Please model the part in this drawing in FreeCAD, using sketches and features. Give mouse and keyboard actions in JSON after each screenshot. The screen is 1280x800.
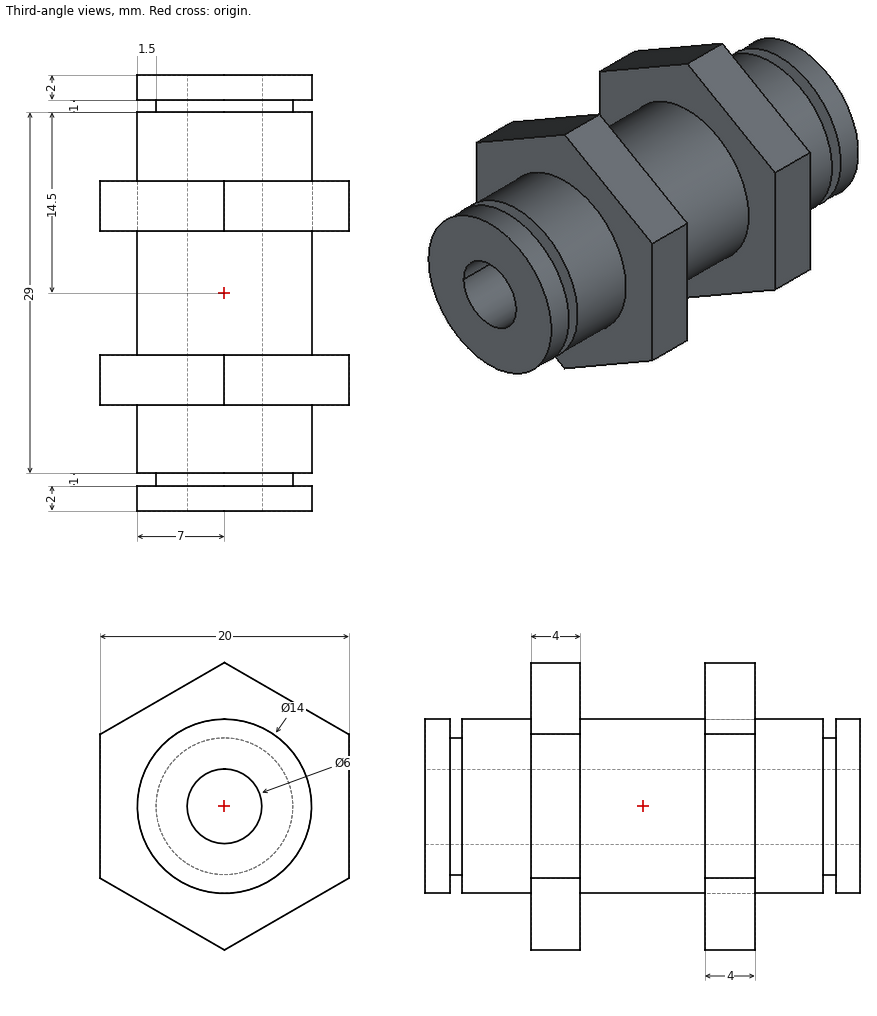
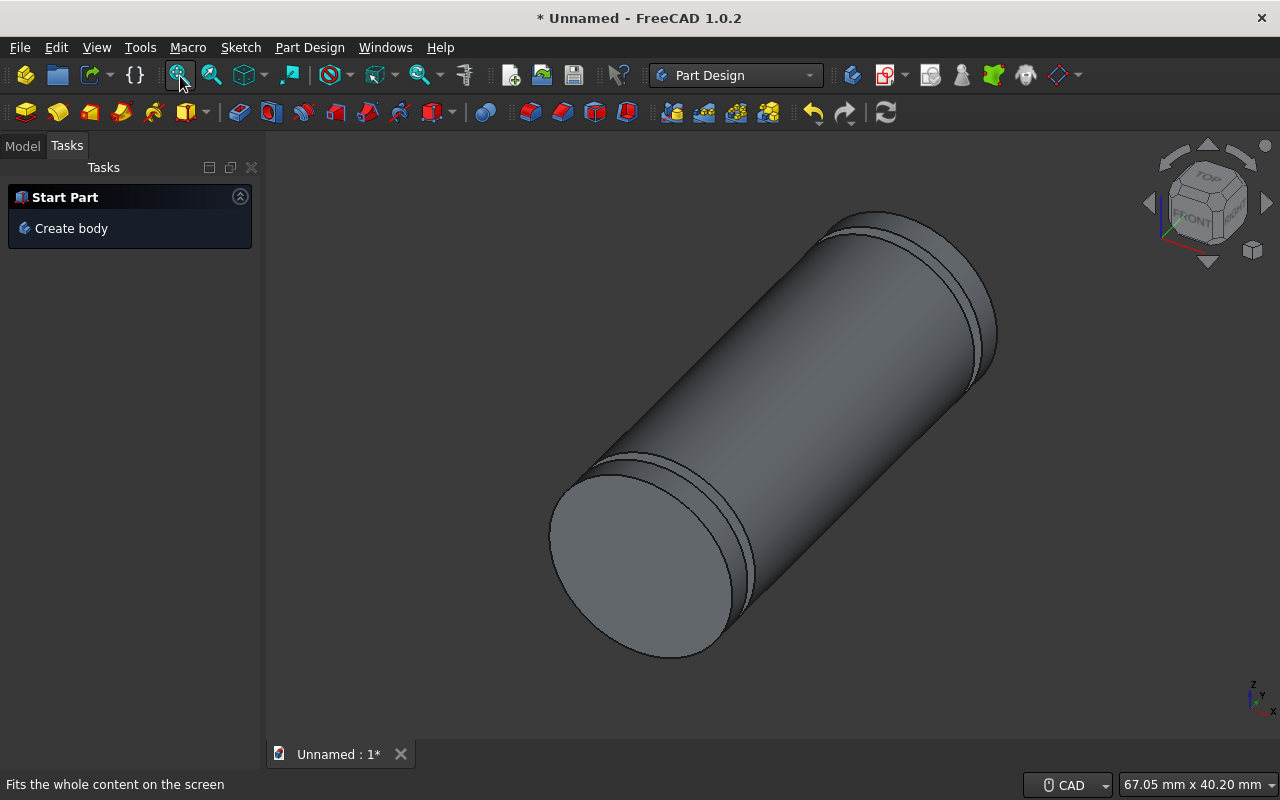
{"action": "key", "text": "4"}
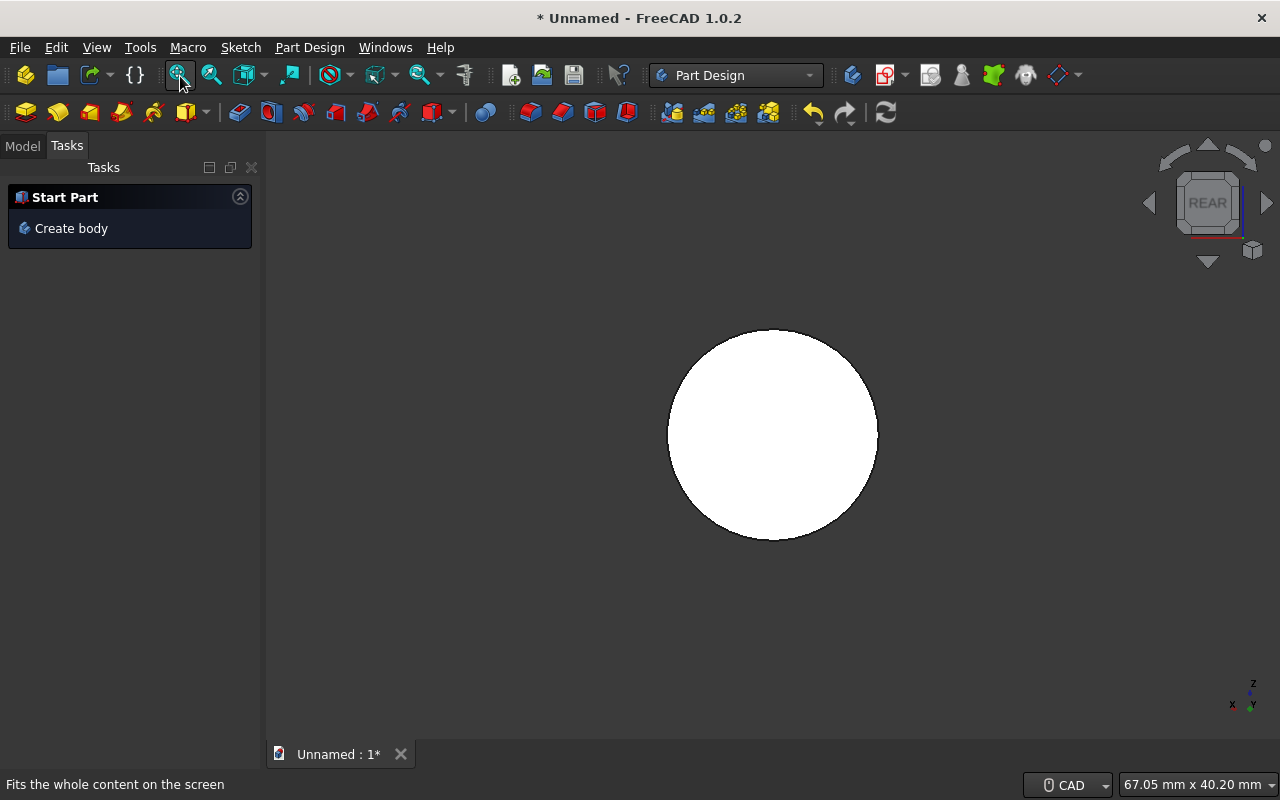
{"action": "left_click", "coordinate": [180, 76]}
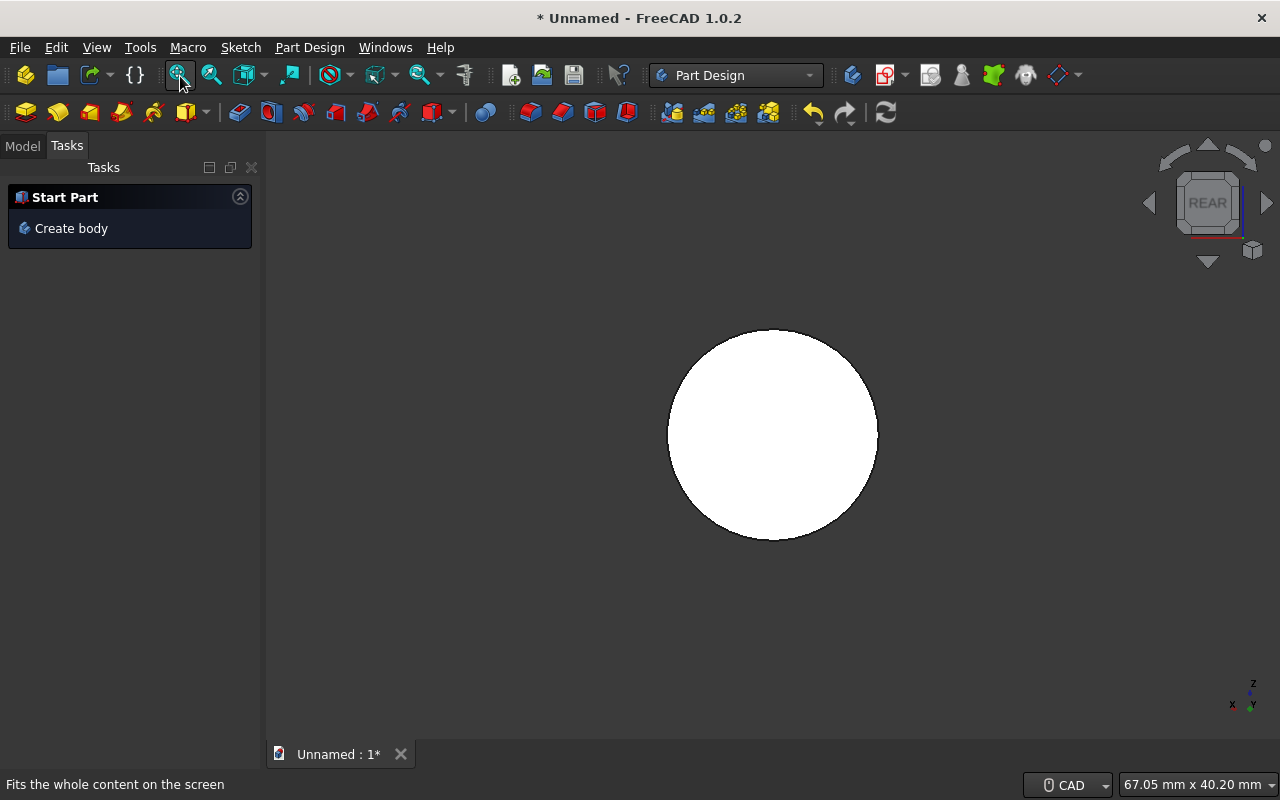
{"action": "left_click", "coordinate": [773, 434]}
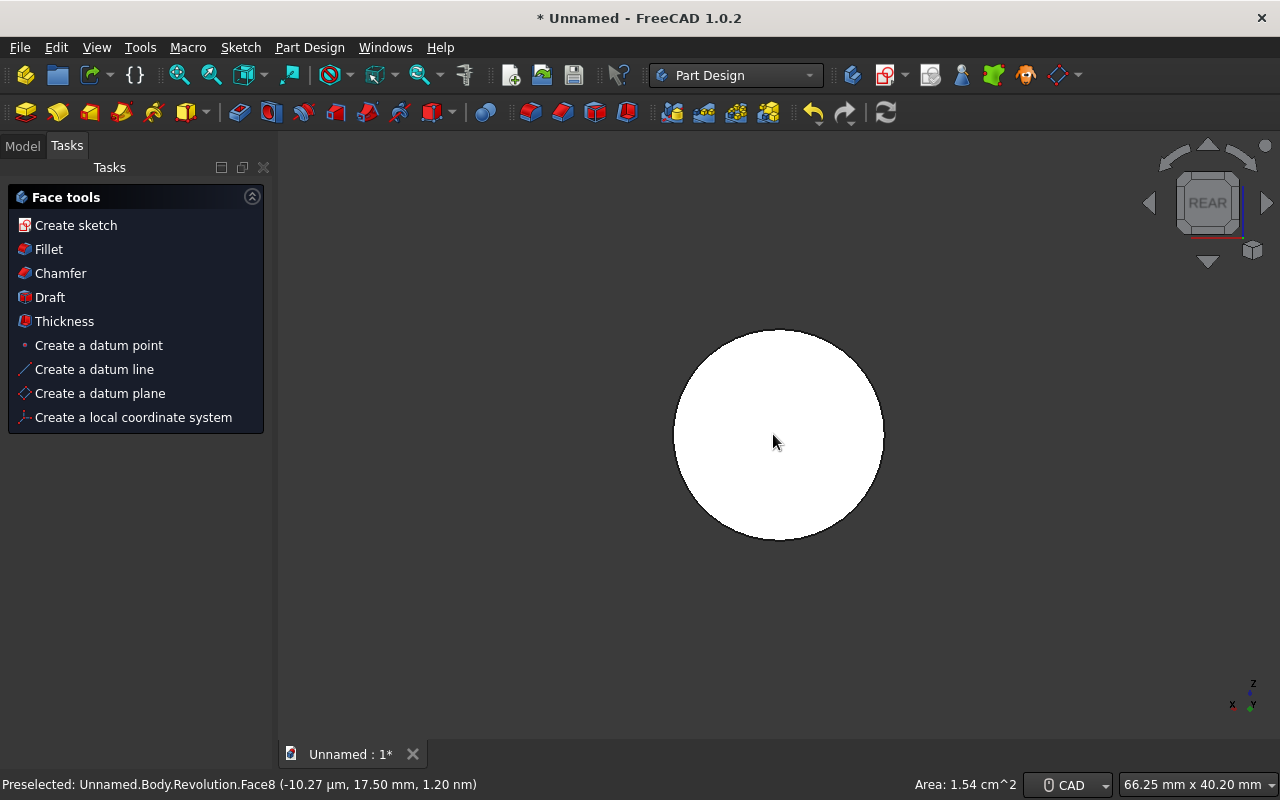
{"action": "left_click", "coordinate": [886, 76]}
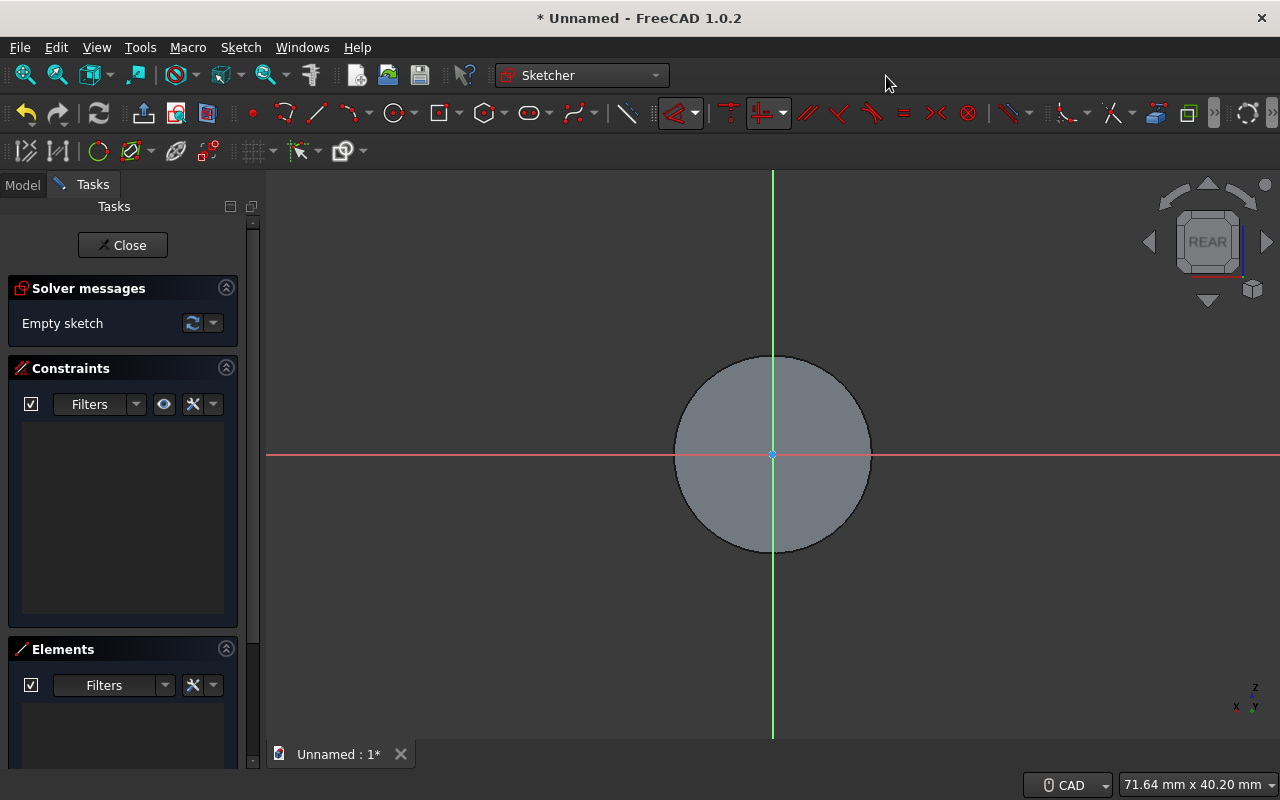
{"action": "scroll", "coordinate": [795, 455], "scroll_direction": "up", "scroll_amount": 7}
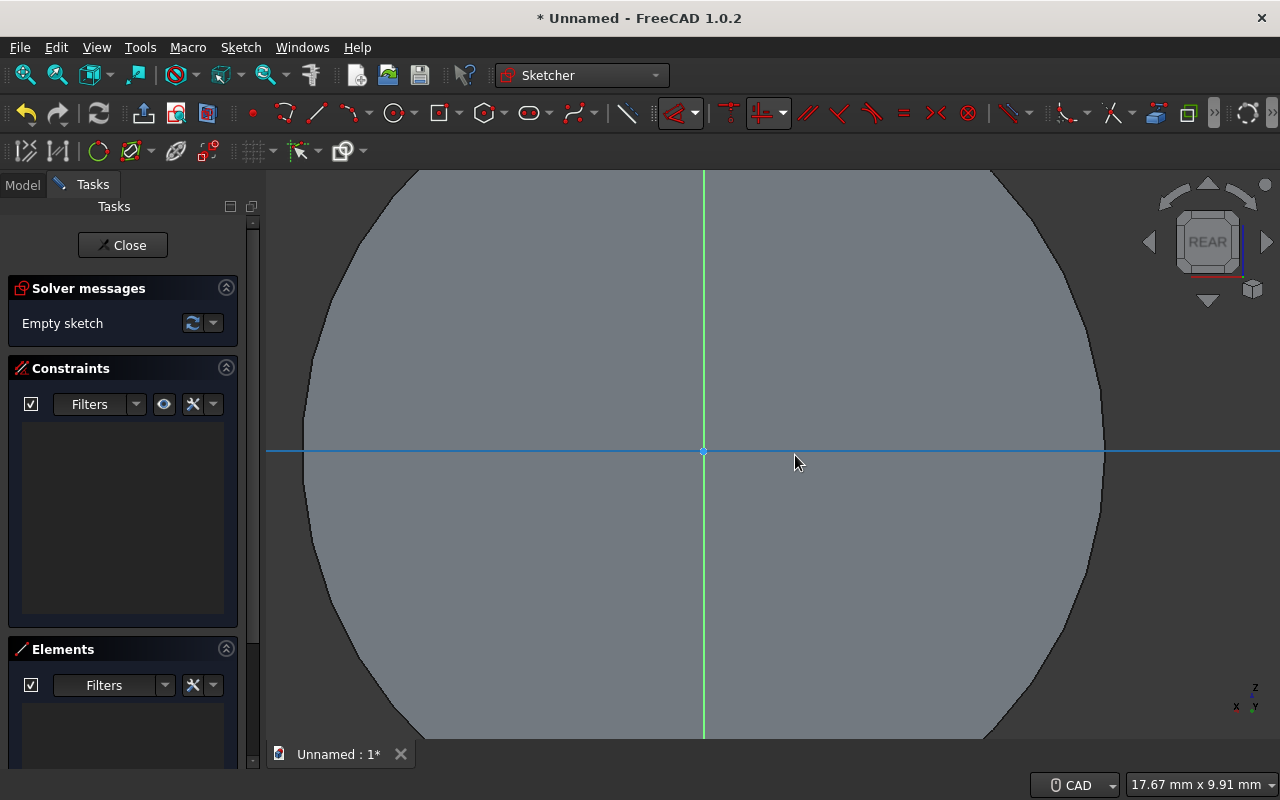
{"action": "left_click", "coordinate": [394, 114]}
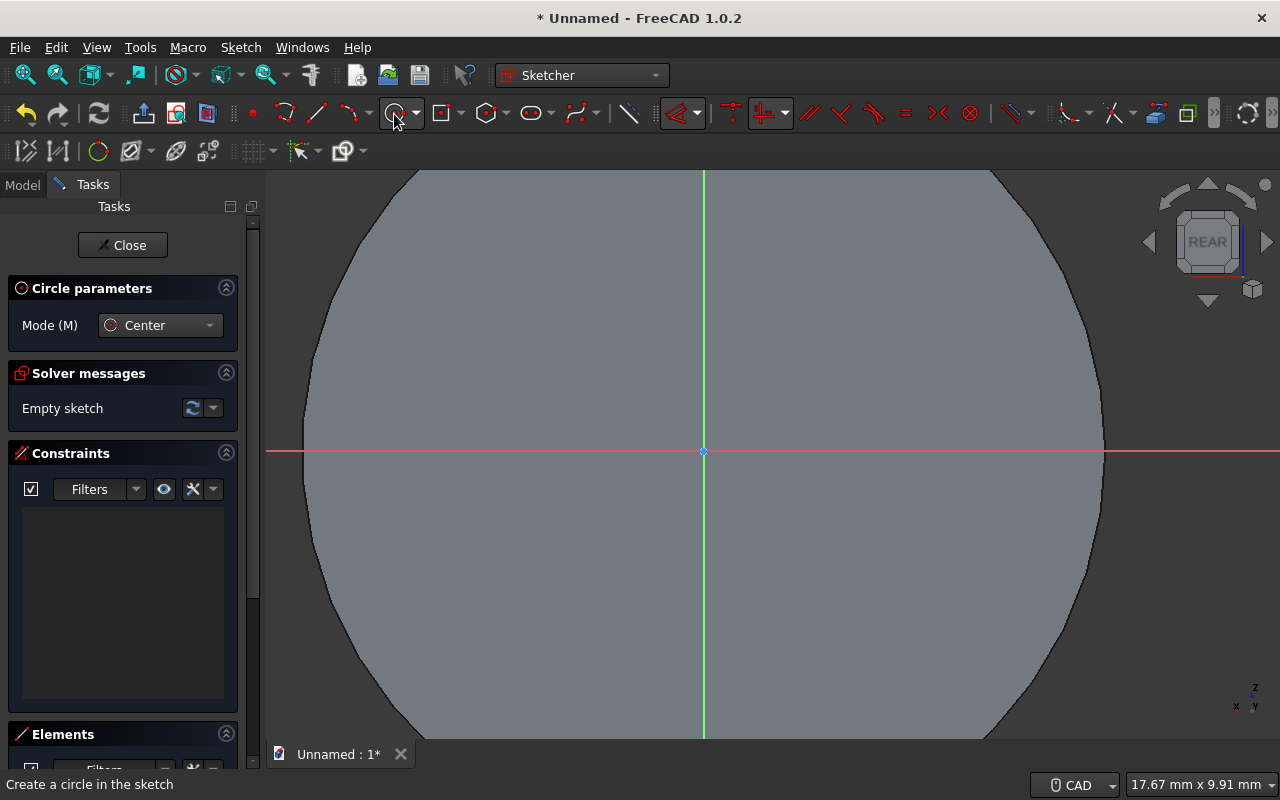
{"action": "left_click", "coordinate": [704, 451]}
{"action": "left_click", "coordinate": [825, 330]}
{"action": "key", "text": "Escape"}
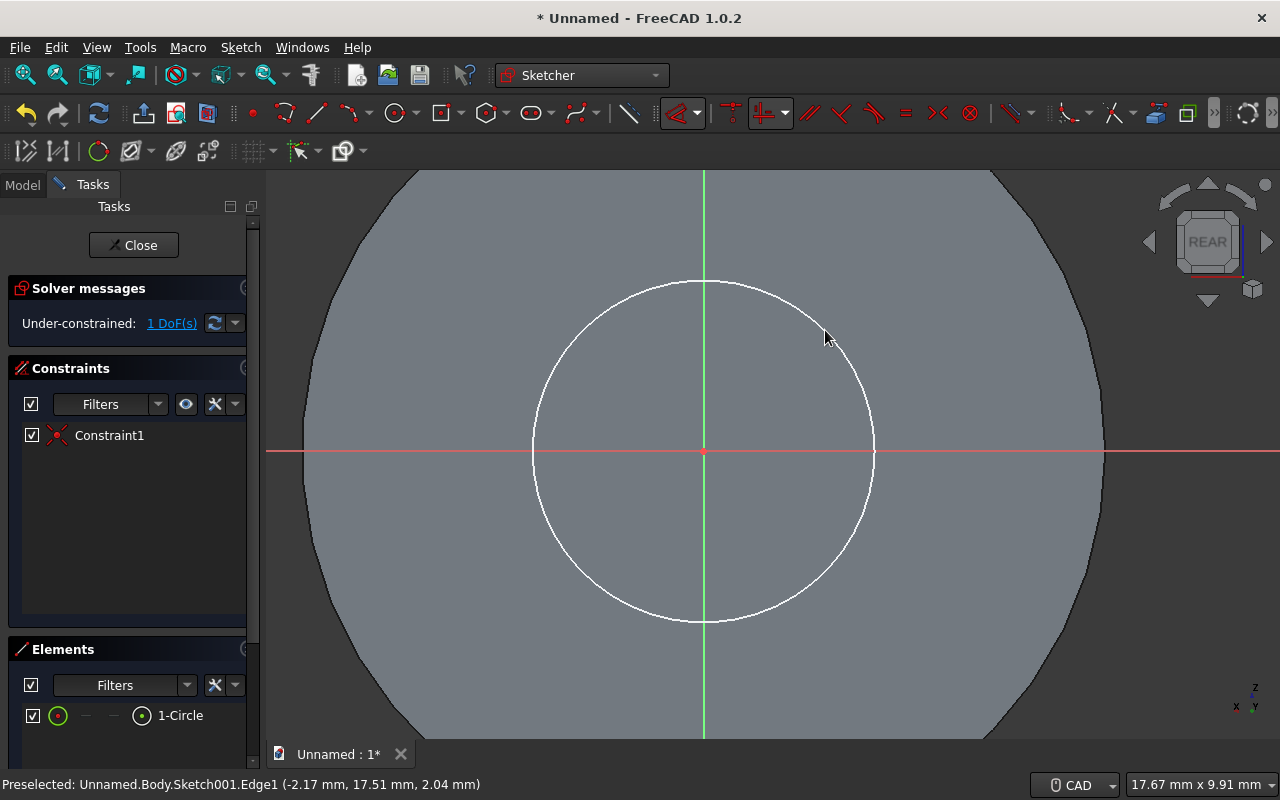
{"action": "left_click", "coordinate": [824, 330]}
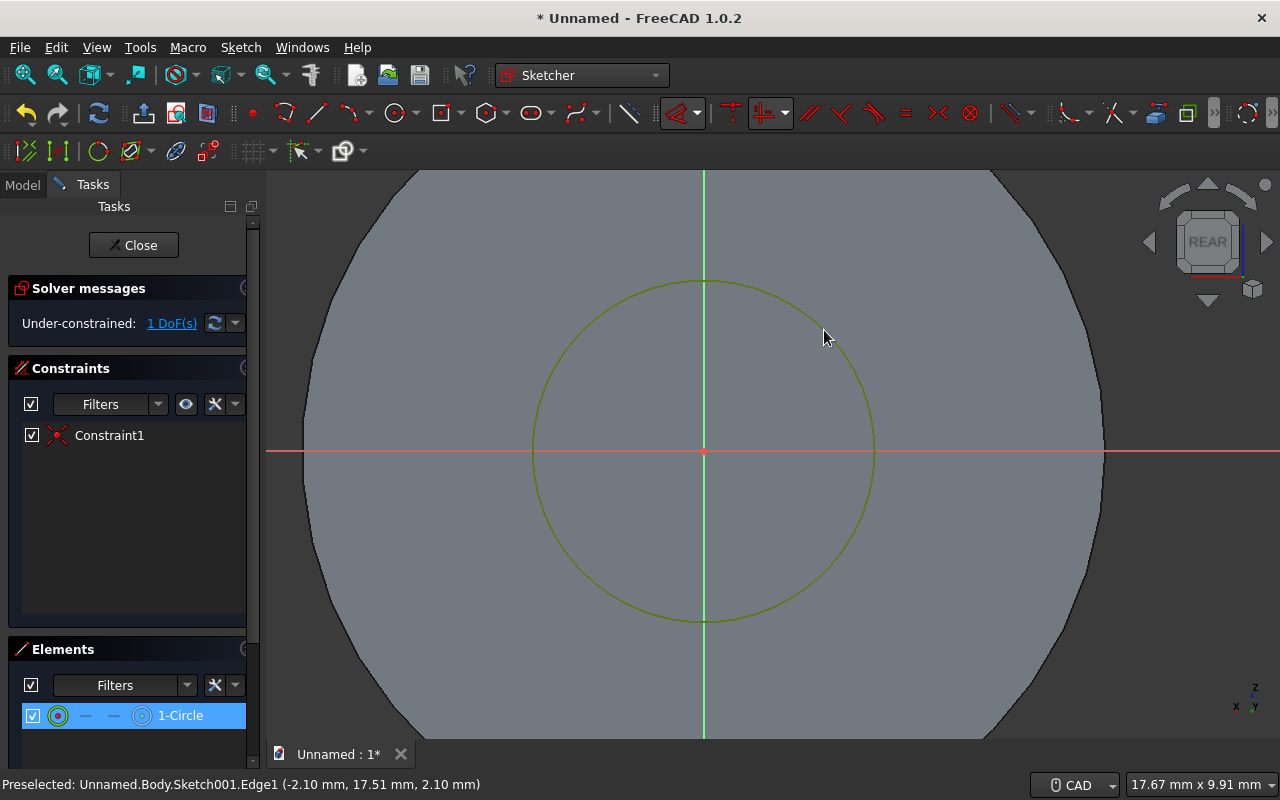
{"action": "left_click", "coordinate": [700, 114]}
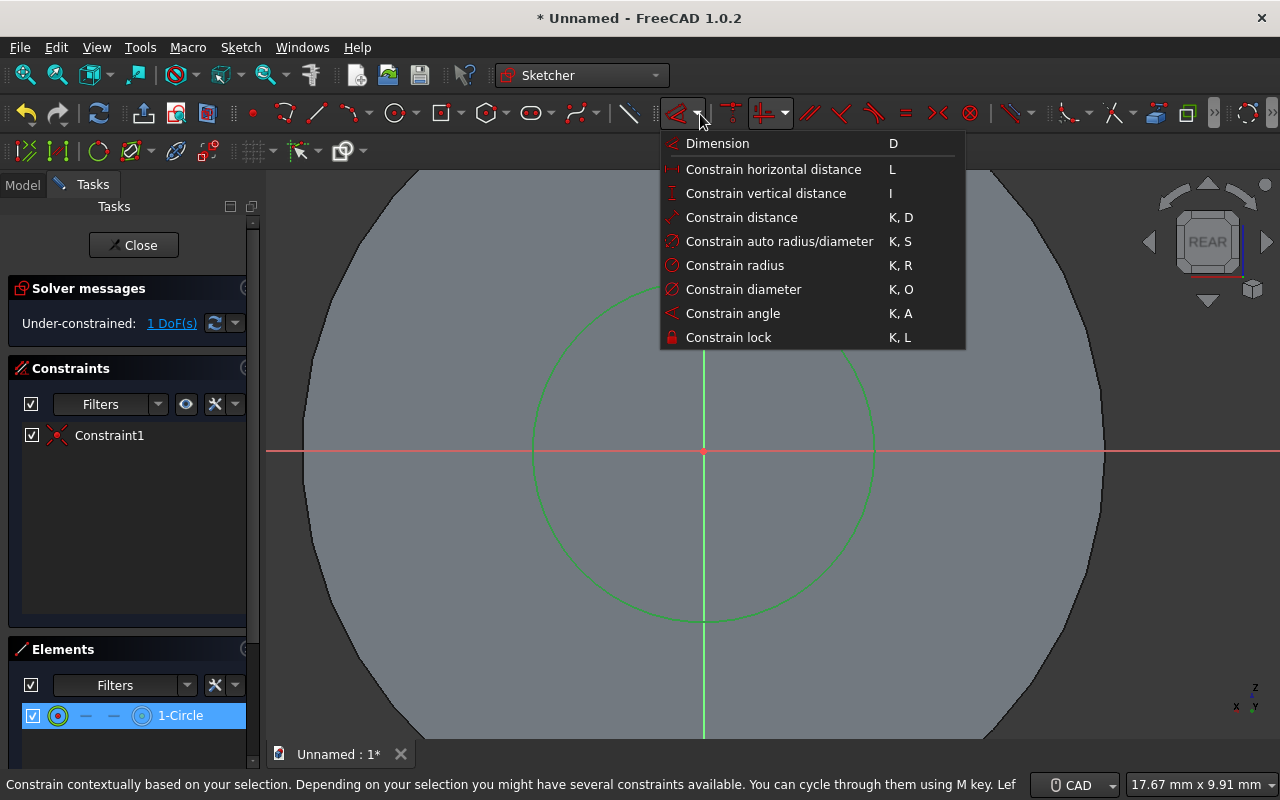
{"action": "left_click", "coordinate": [813, 289]}